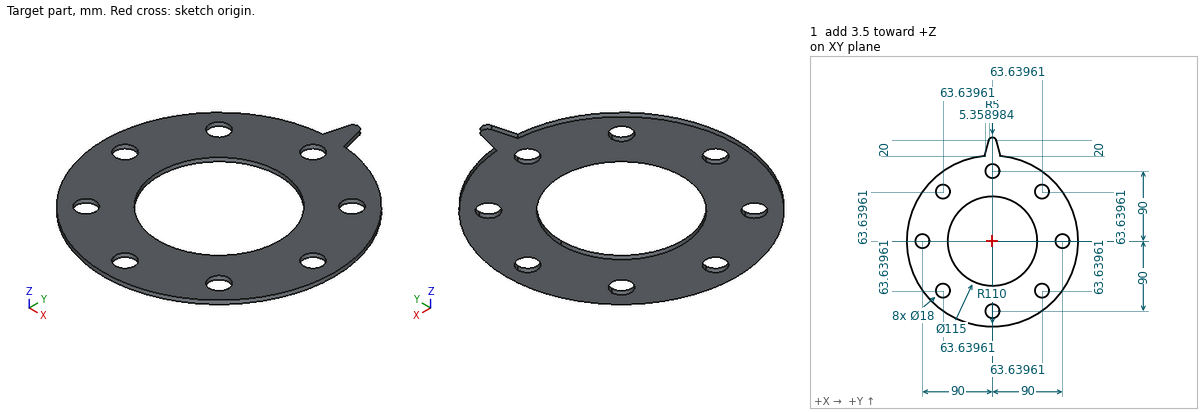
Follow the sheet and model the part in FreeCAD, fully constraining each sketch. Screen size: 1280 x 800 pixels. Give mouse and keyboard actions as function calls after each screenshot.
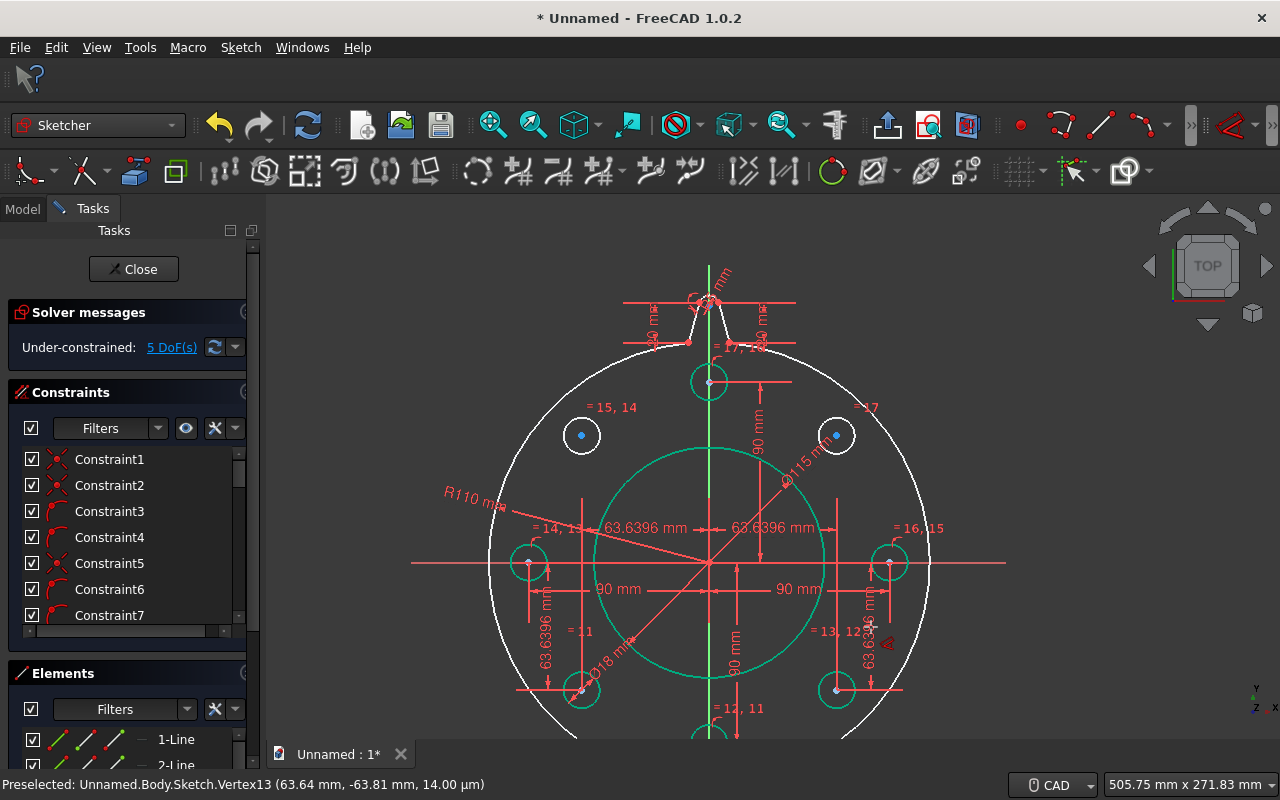
click(582, 436)
click(646, 402)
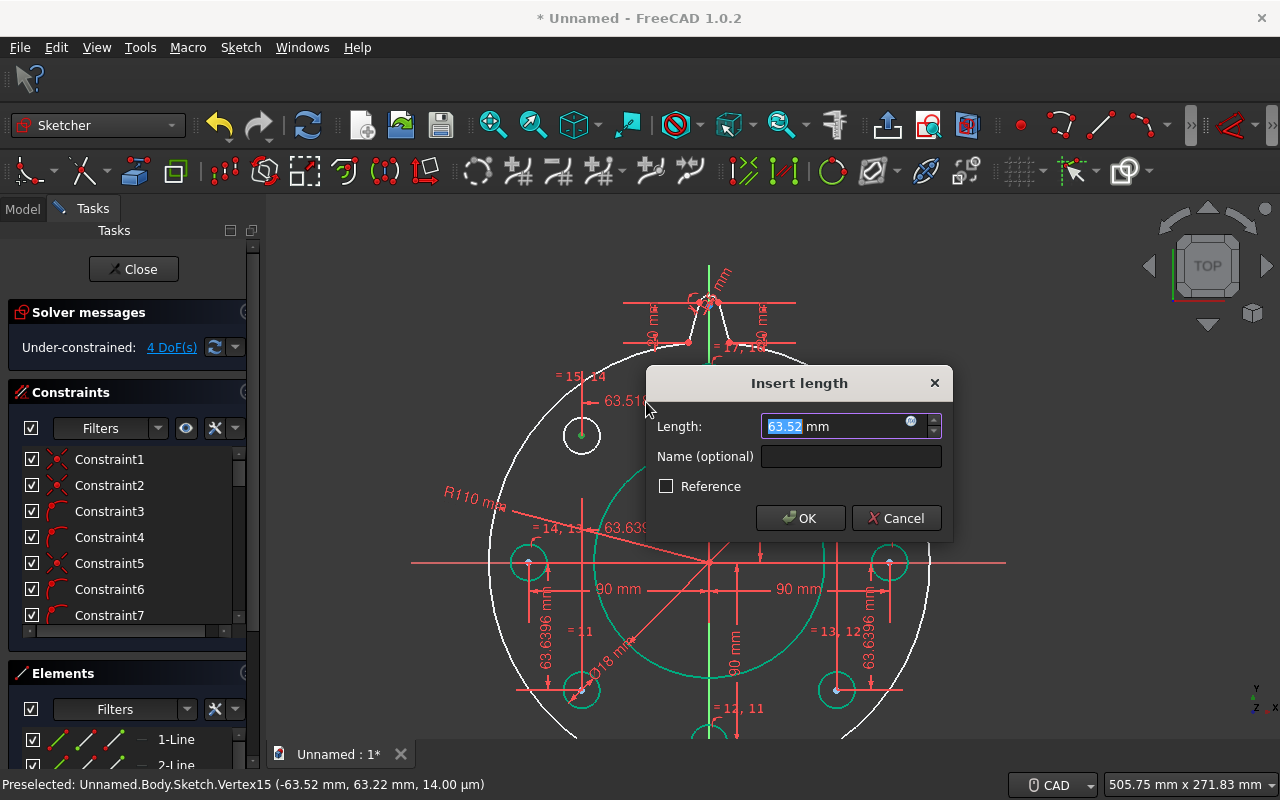
text(63.63961)
key(Return)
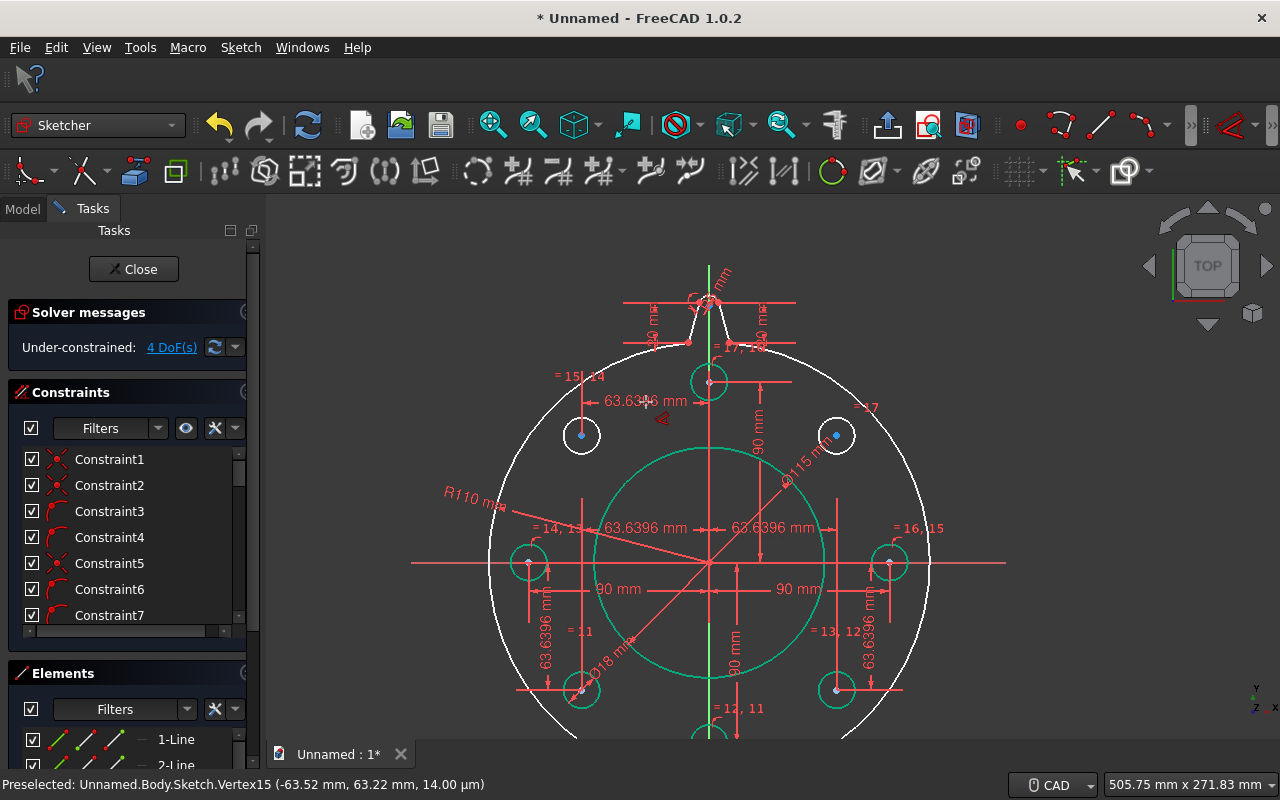
click(582, 436)
click(548, 499)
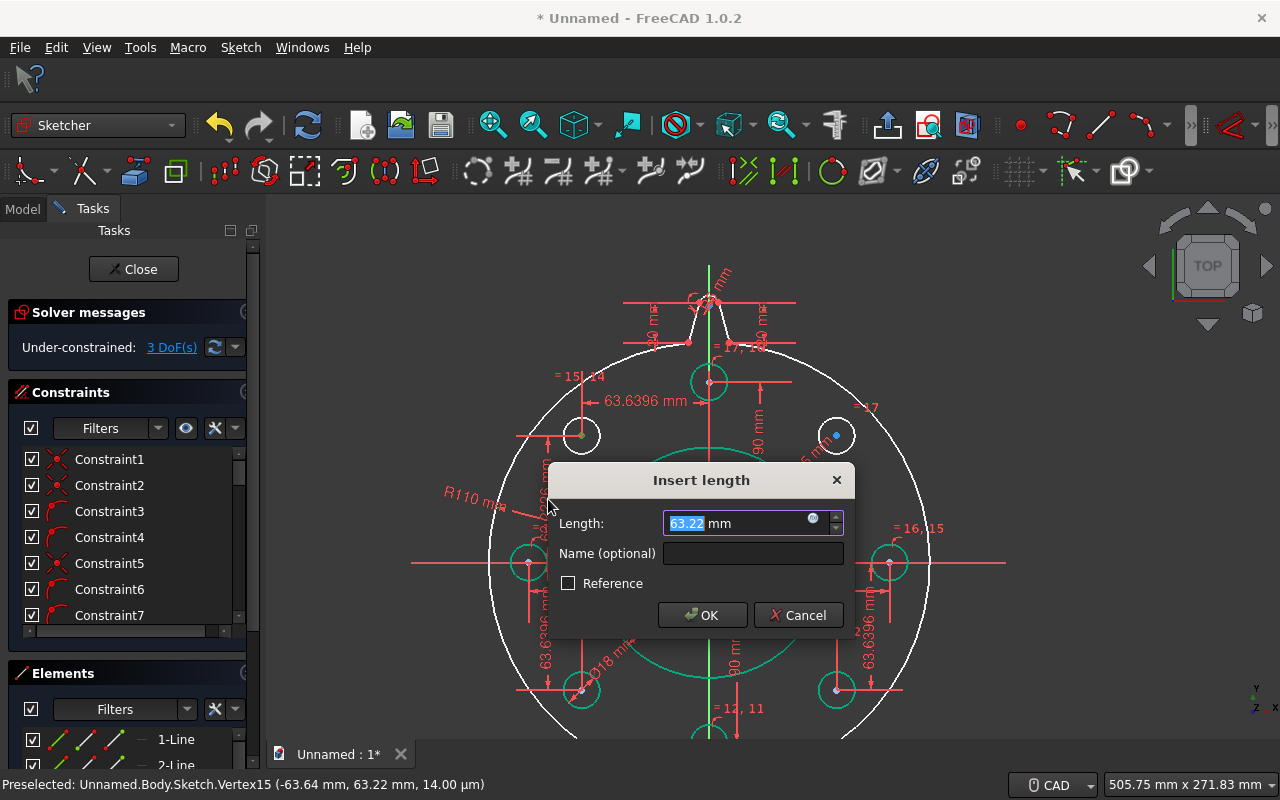
text(63.63961)
key(Return)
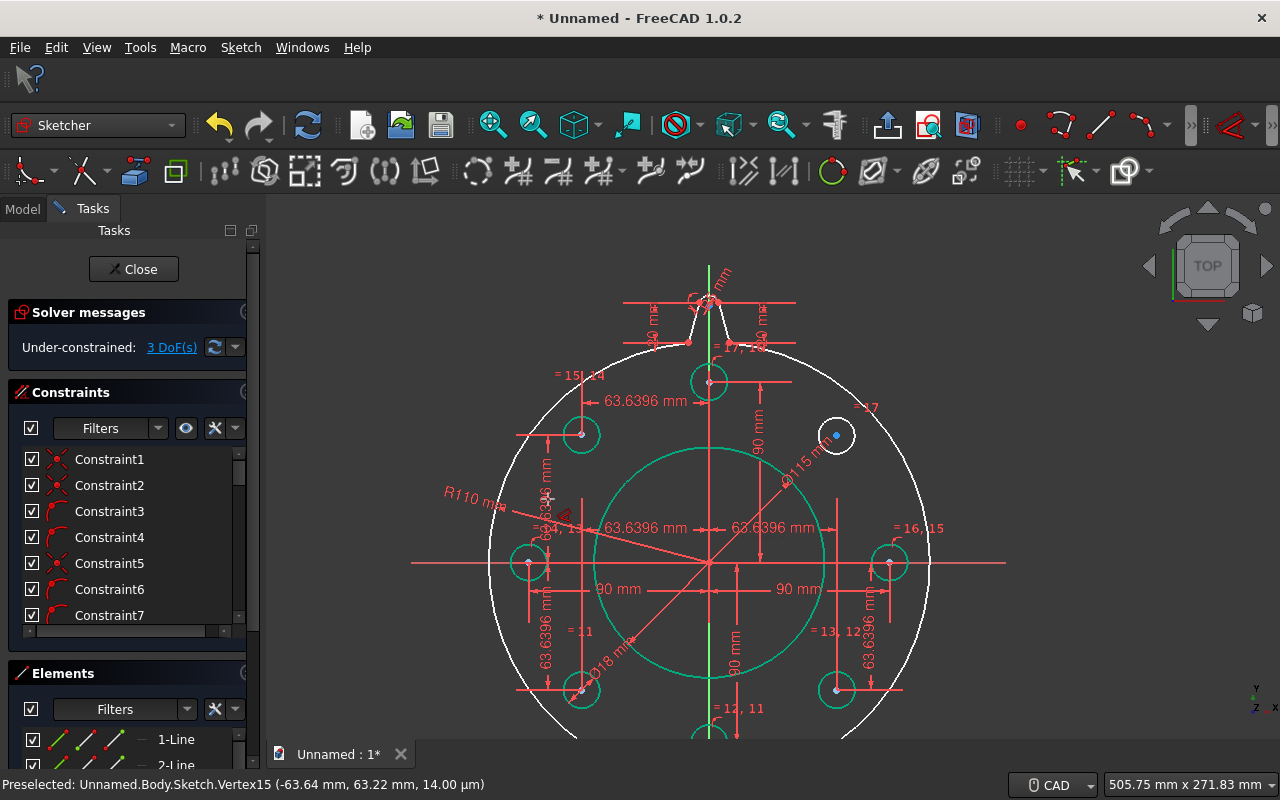
click(837, 436)
click(773, 402)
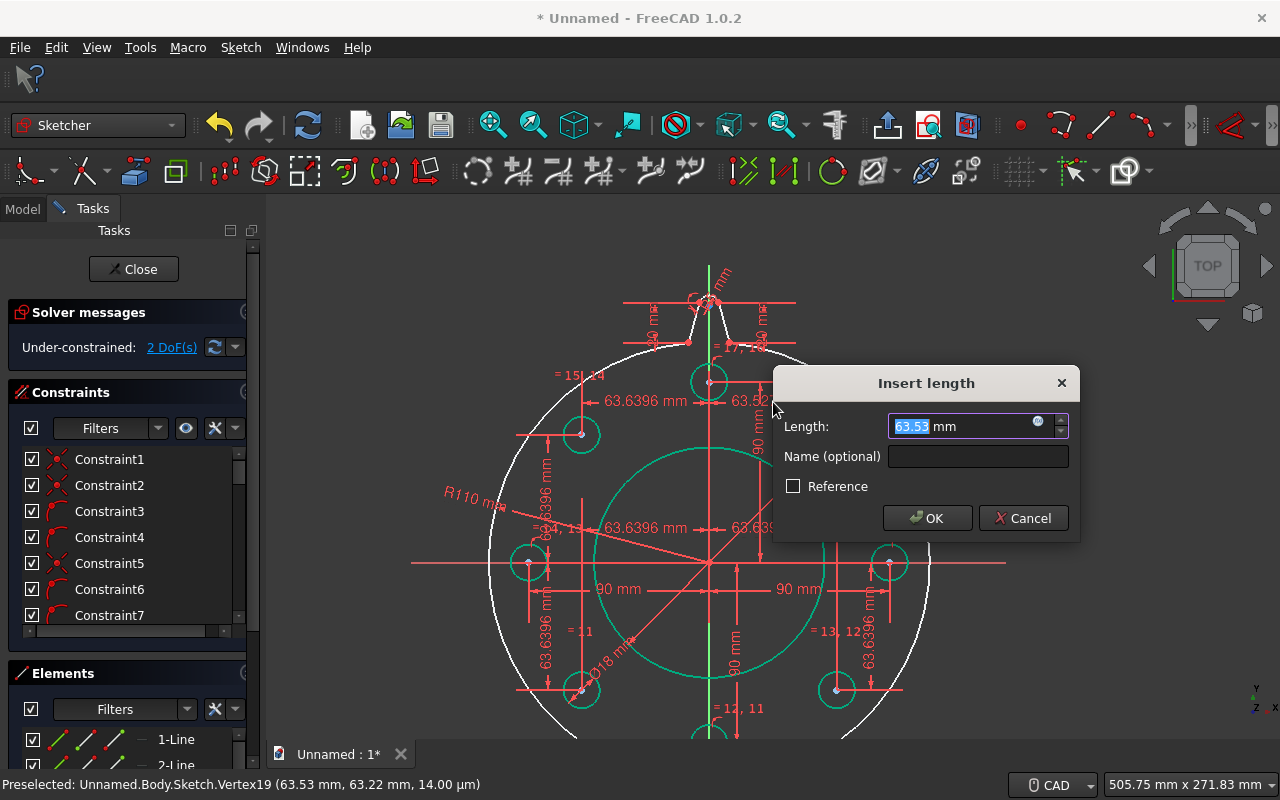
text(63.63961)
key(Return)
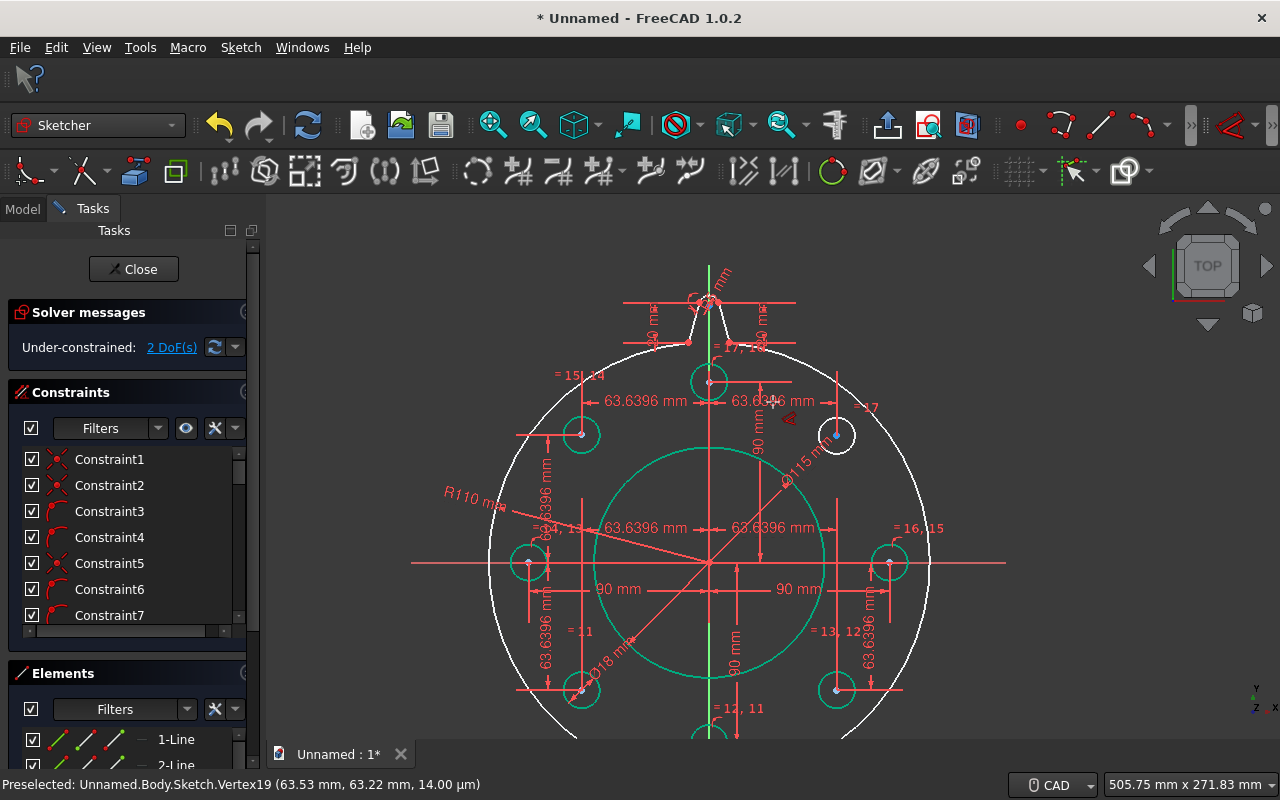
click(837, 436)
click(871, 499)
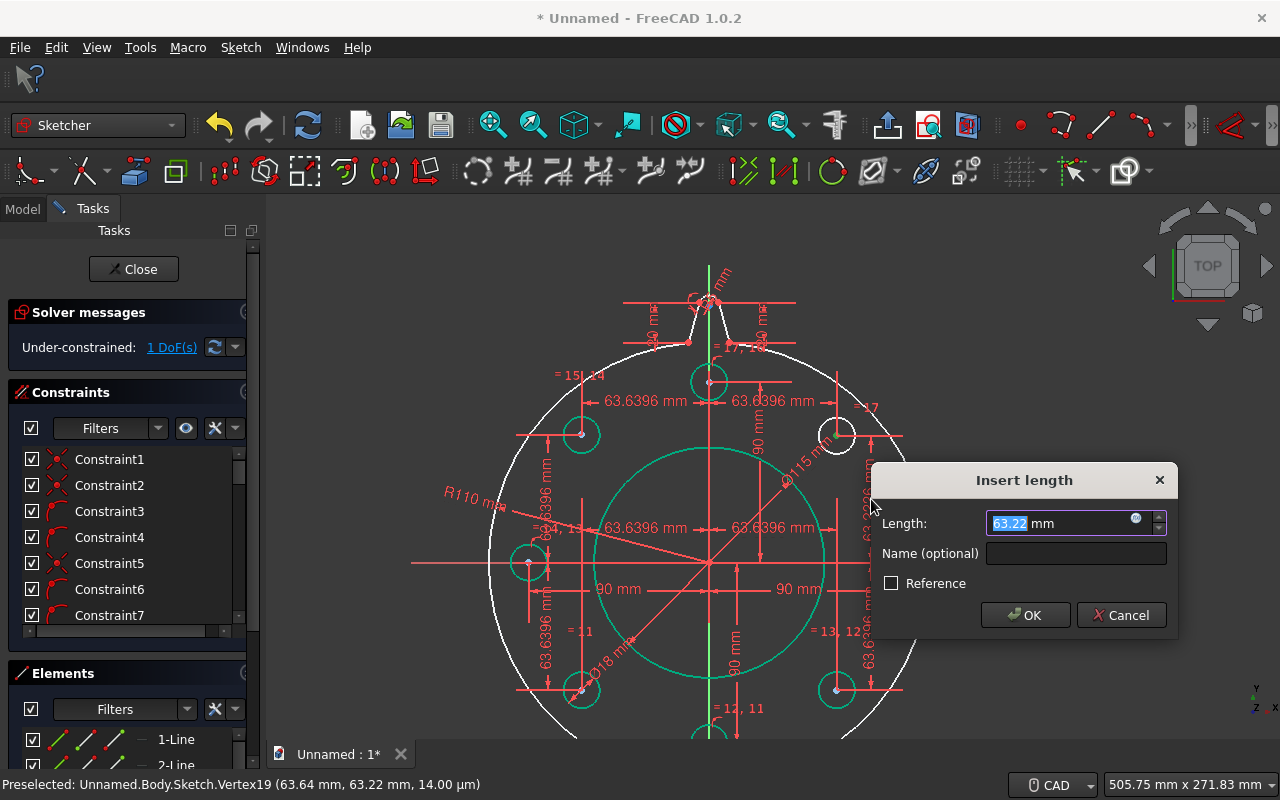
text(63.63961)
key(Return)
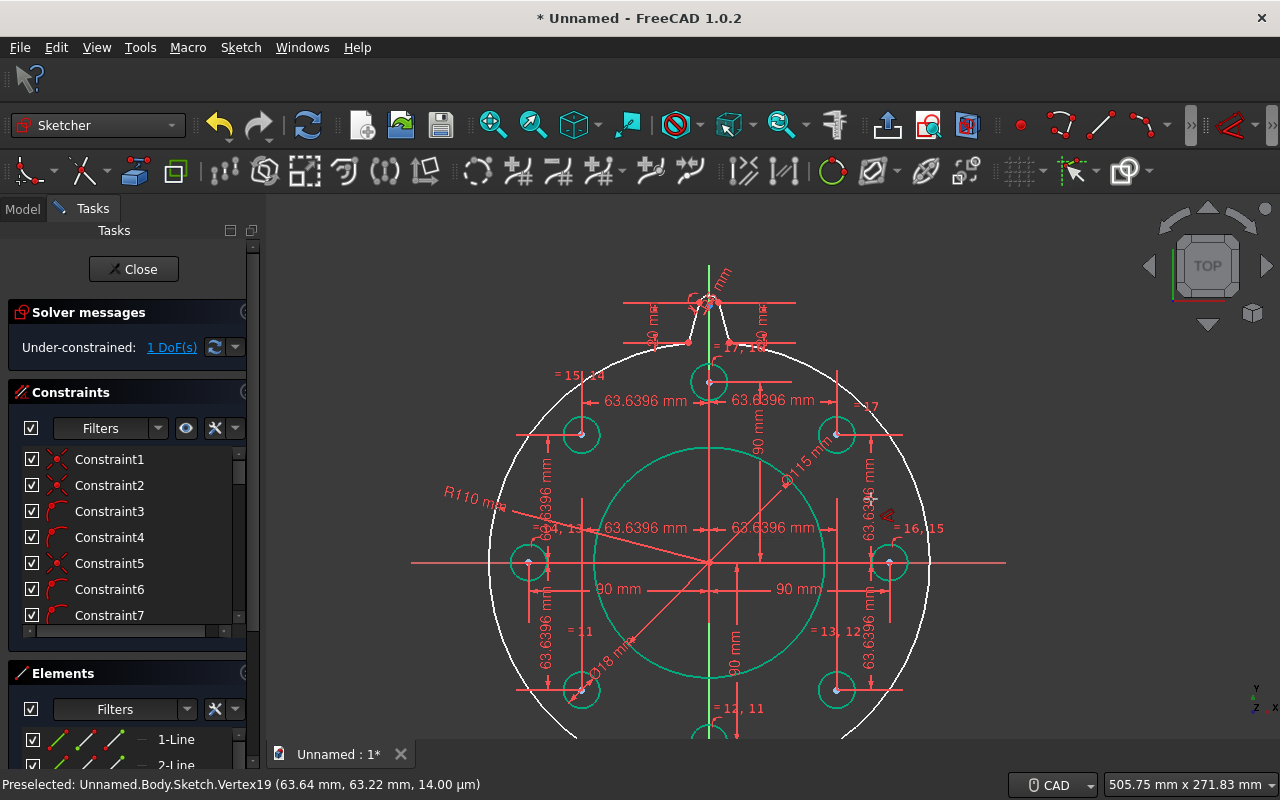
scroll(696, 315, up, 7)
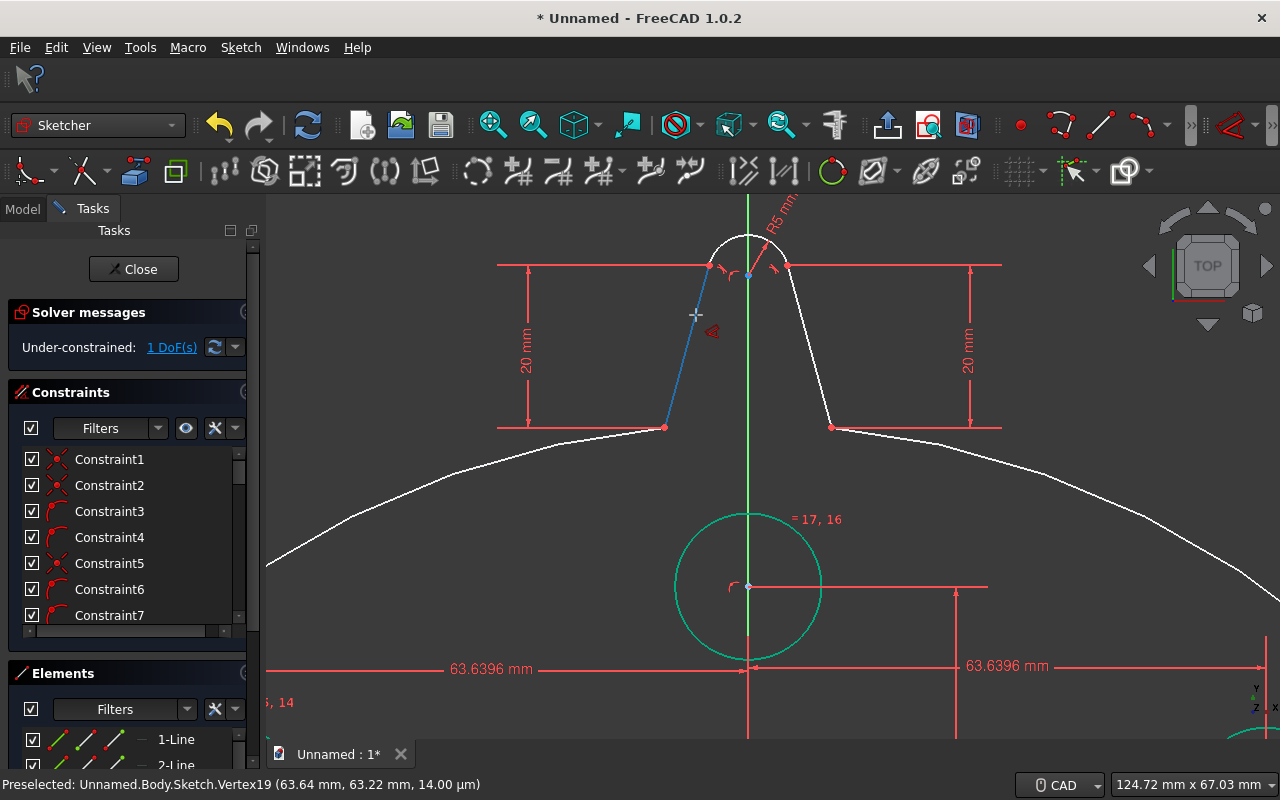
click(696, 314)
click(687, 231)